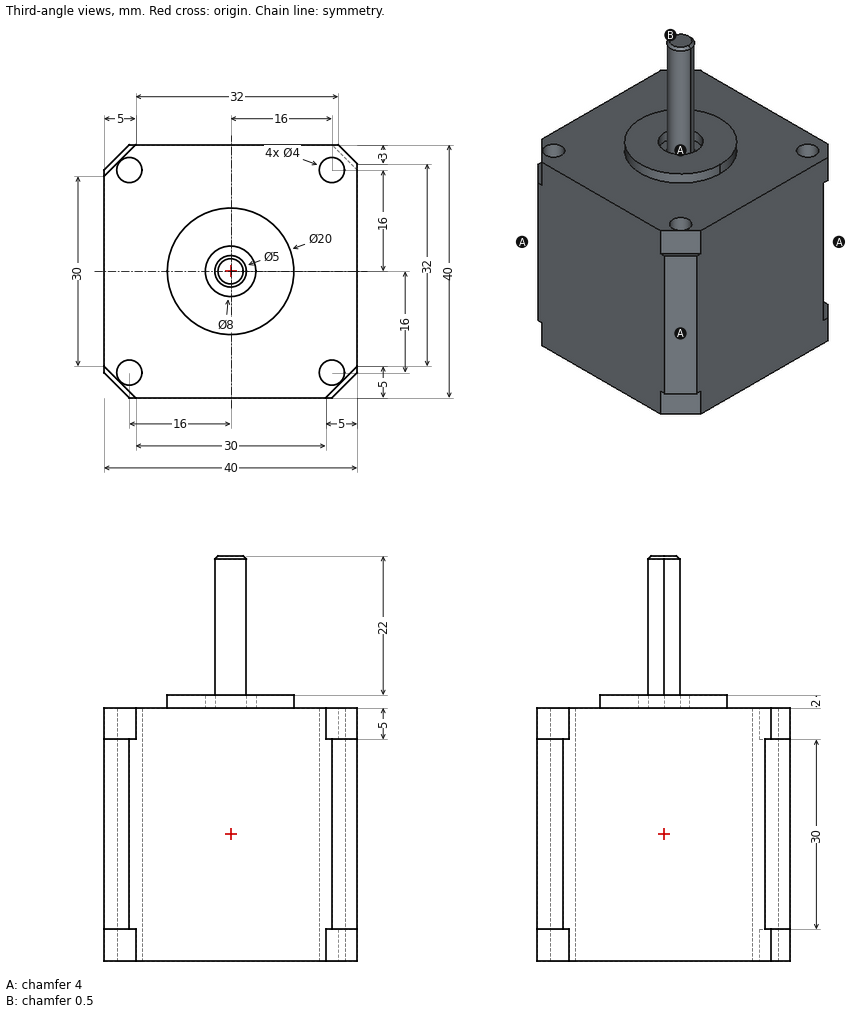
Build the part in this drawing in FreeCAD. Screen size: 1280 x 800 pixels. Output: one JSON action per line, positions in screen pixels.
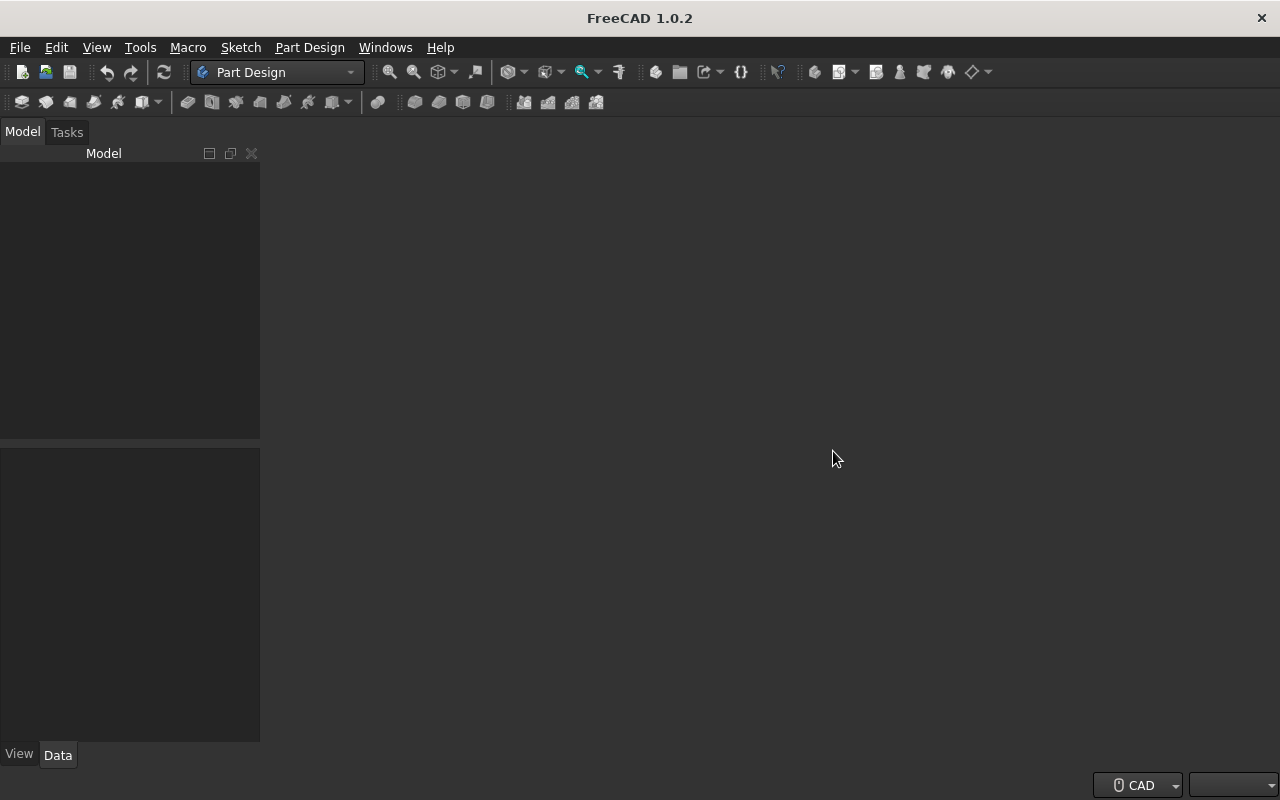
{"action": "left_click", "coordinate": [22, 72]}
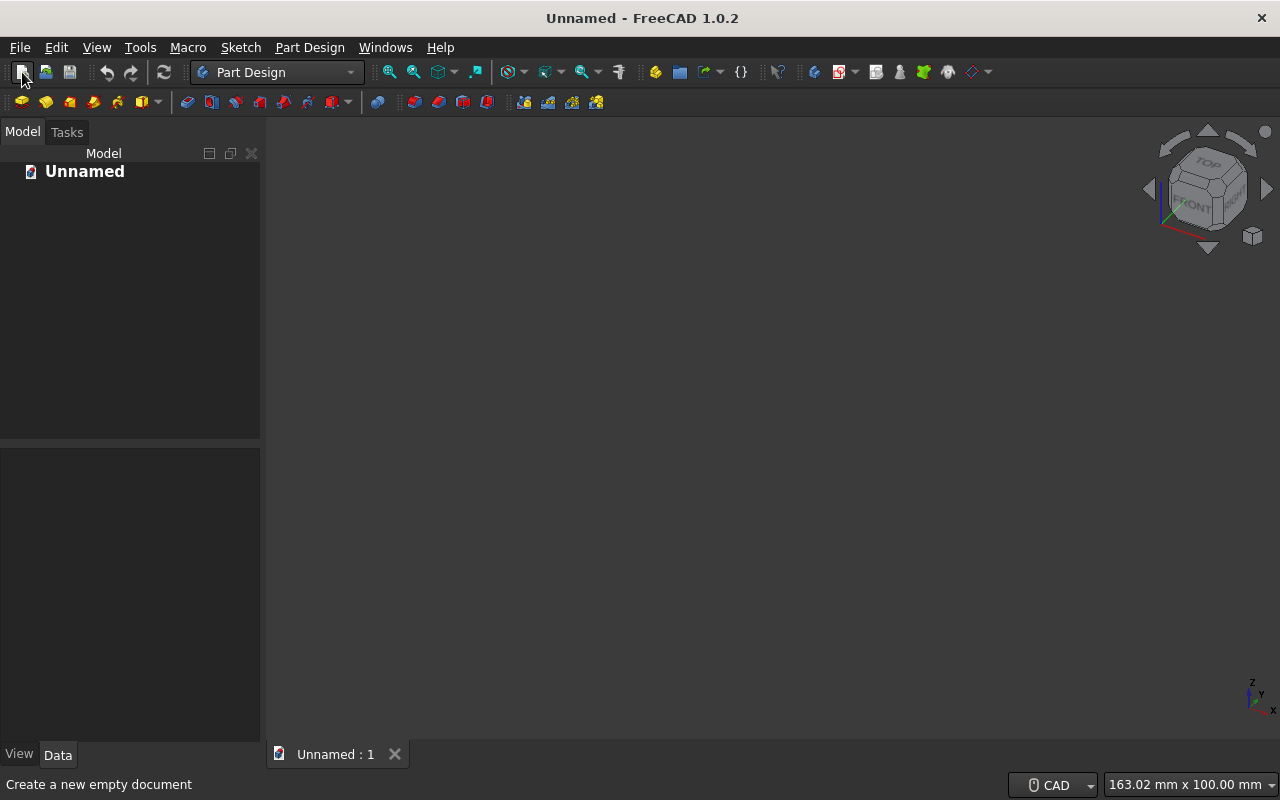
{"action": "left_click", "coordinate": [840, 72]}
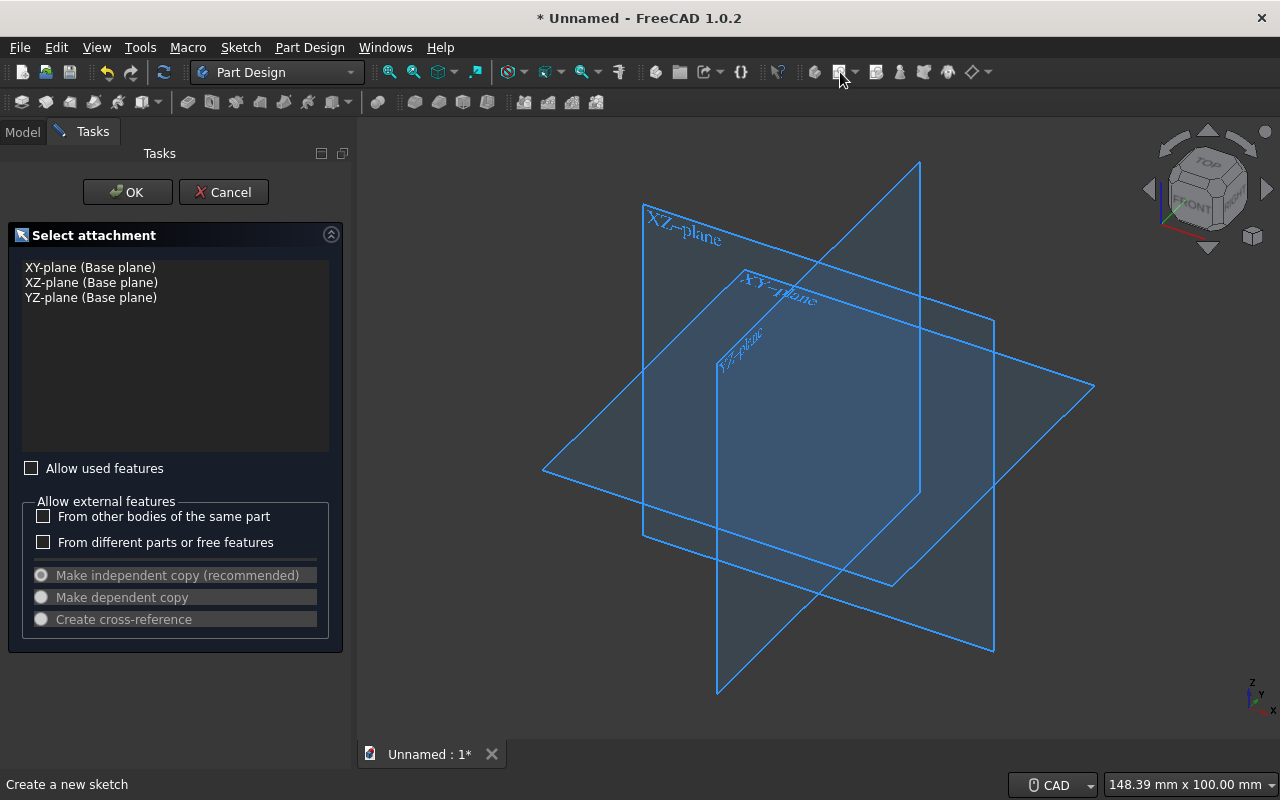
{"action": "left_click", "coordinate": [82, 268]}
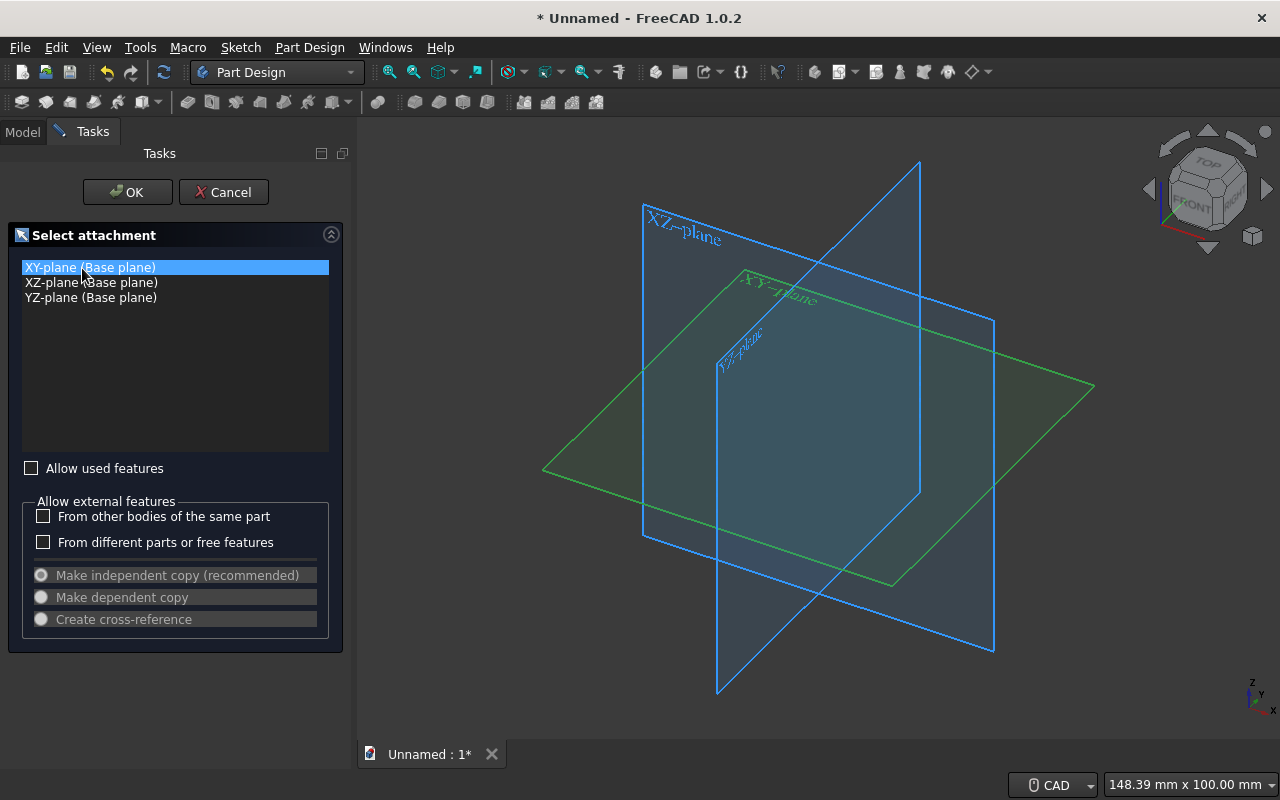
{"action": "left_click", "coordinate": [128, 192]}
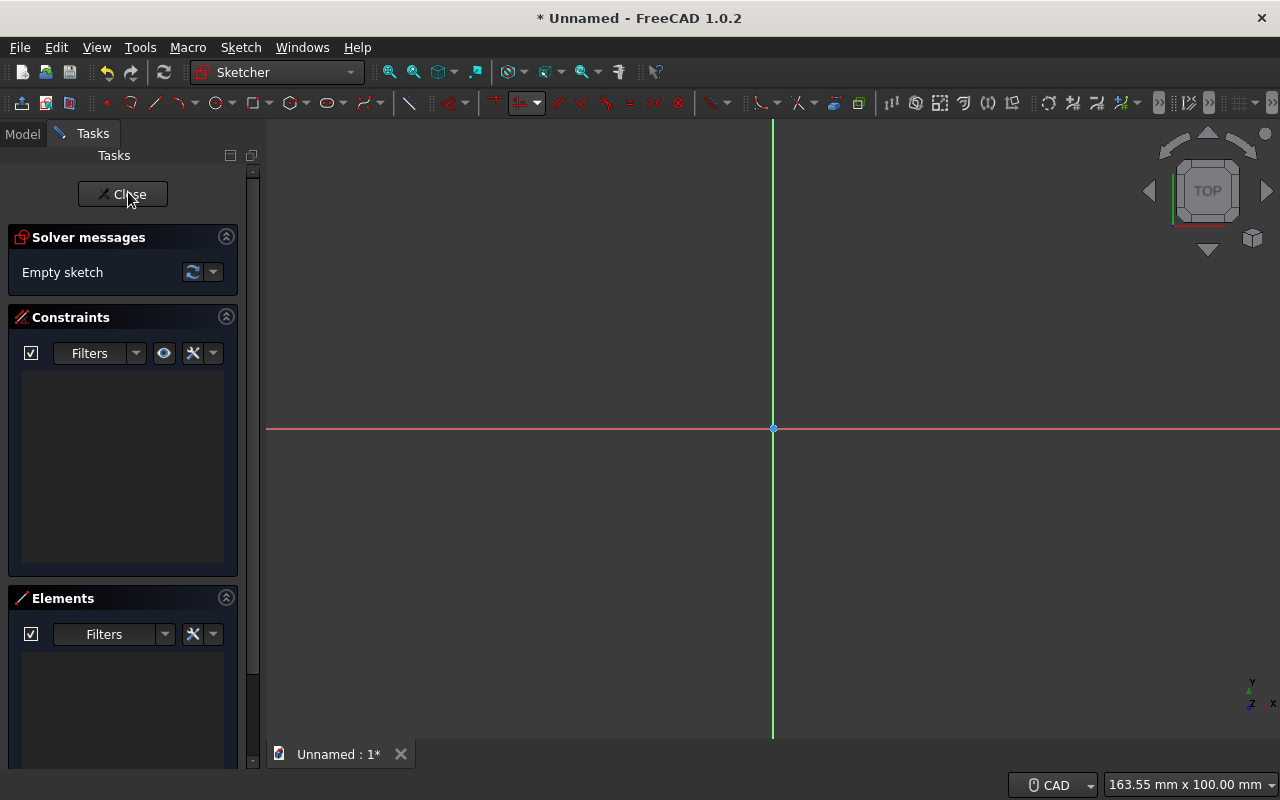
{"action": "scroll", "coordinate": [912, 429], "scroll_direction": "up", "scroll_amount": 2}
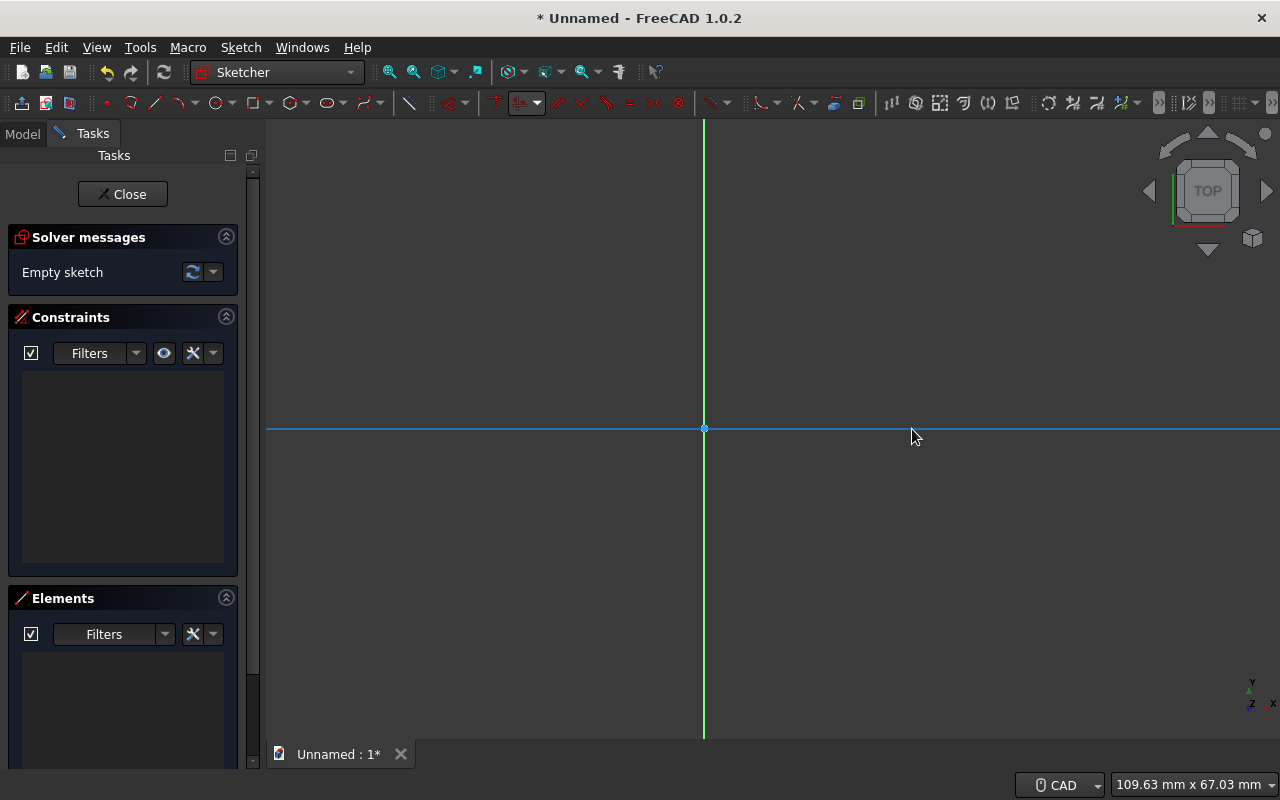
{"action": "key", "text": "g v"}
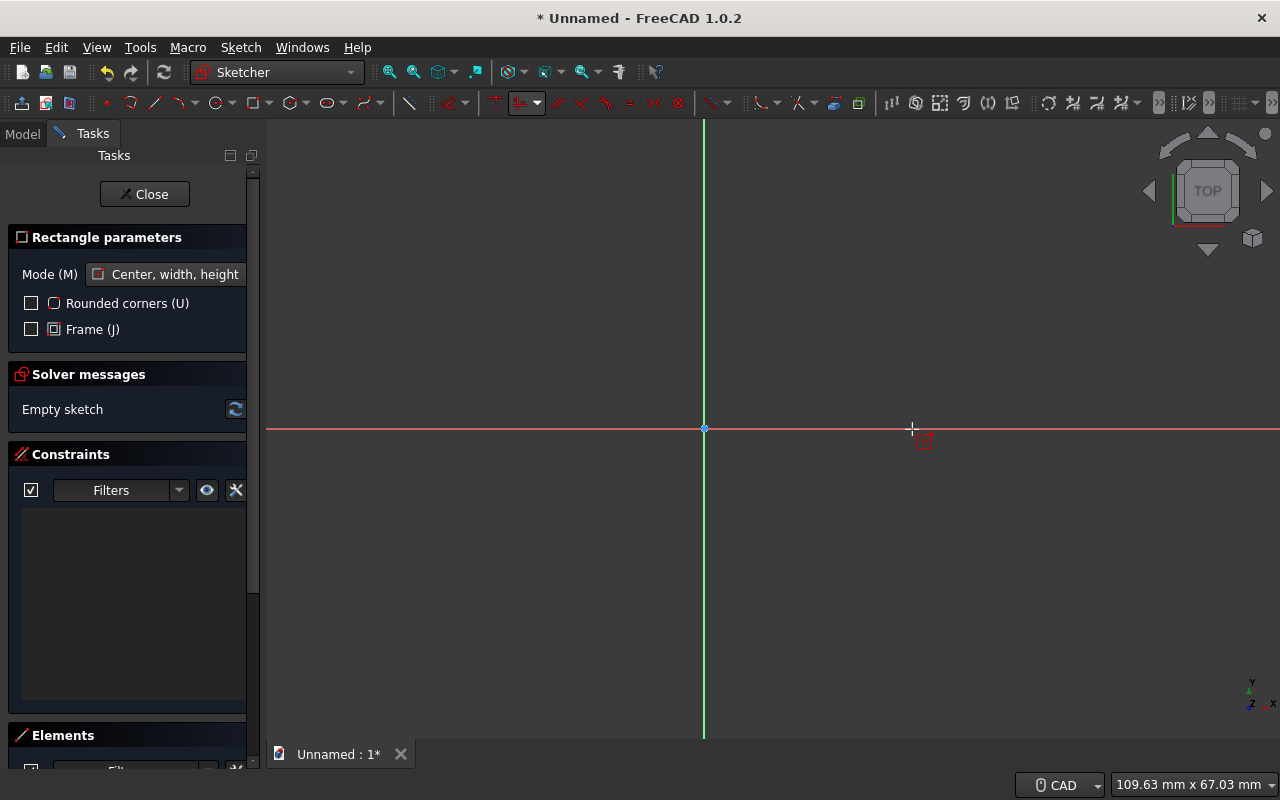
{"action": "left_click", "coordinate": [704, 429]}
{"action": "mouse_move", "coordinate": [889, 244]}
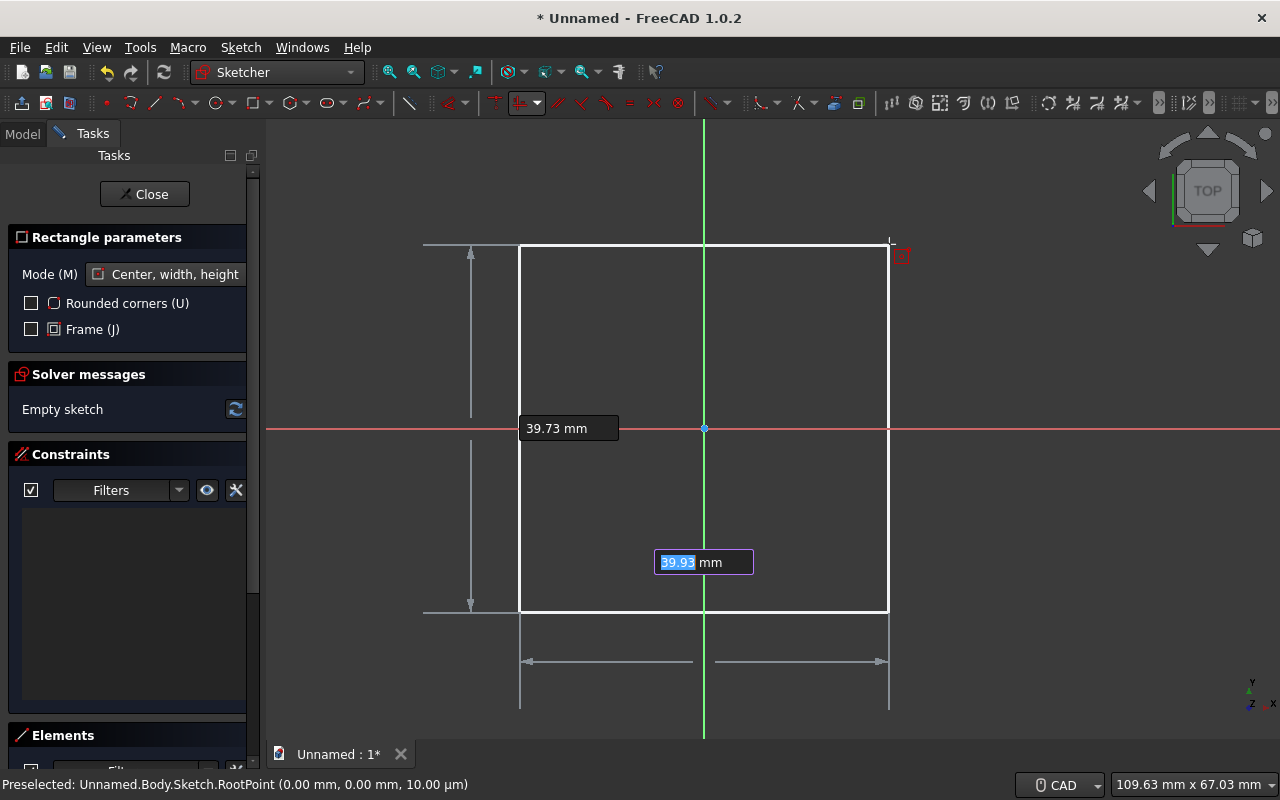
{"action": "type", "text": "40"}
{"action": "key", "text": "Tab"}
{"action": "type", "text": "40"}
{"action": "key", "text": "Return"}
{"action": "key", "text": "Escape"}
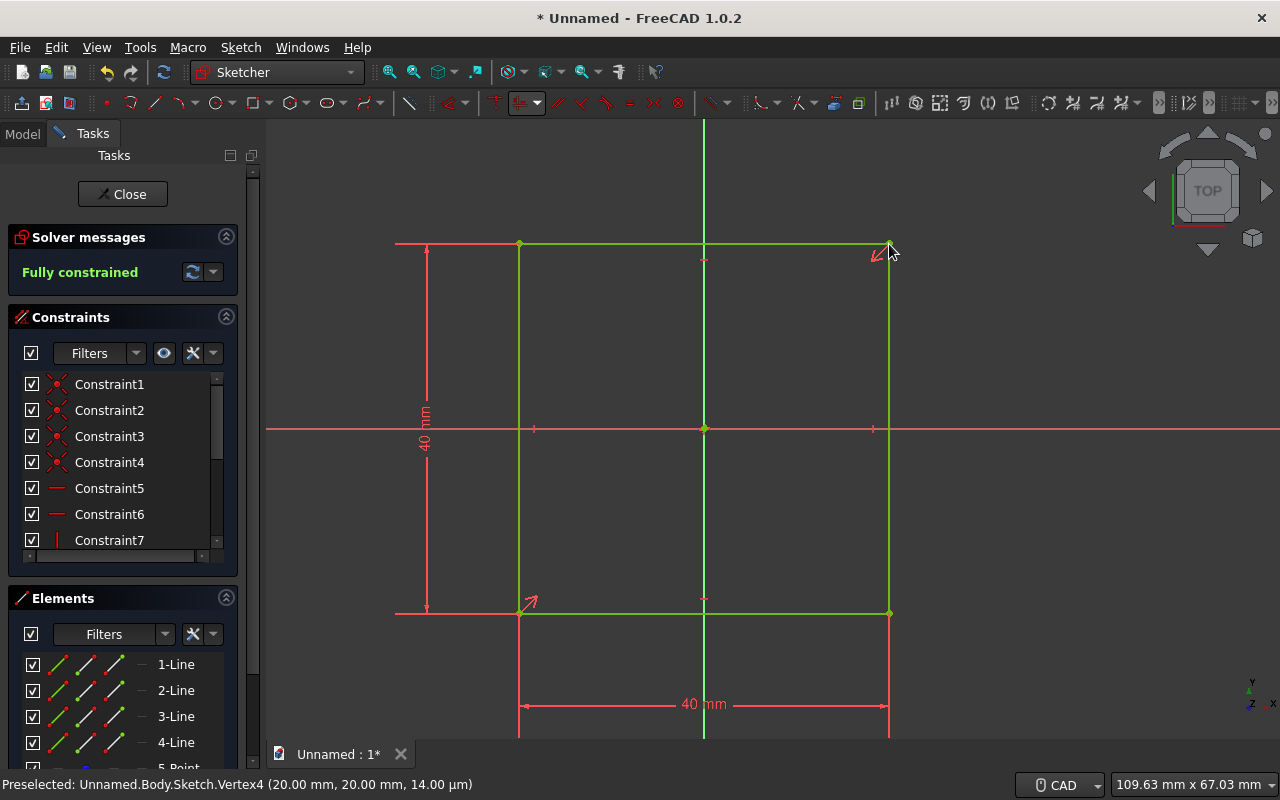
{"action": "left_click", "coordinate": [123, 194]}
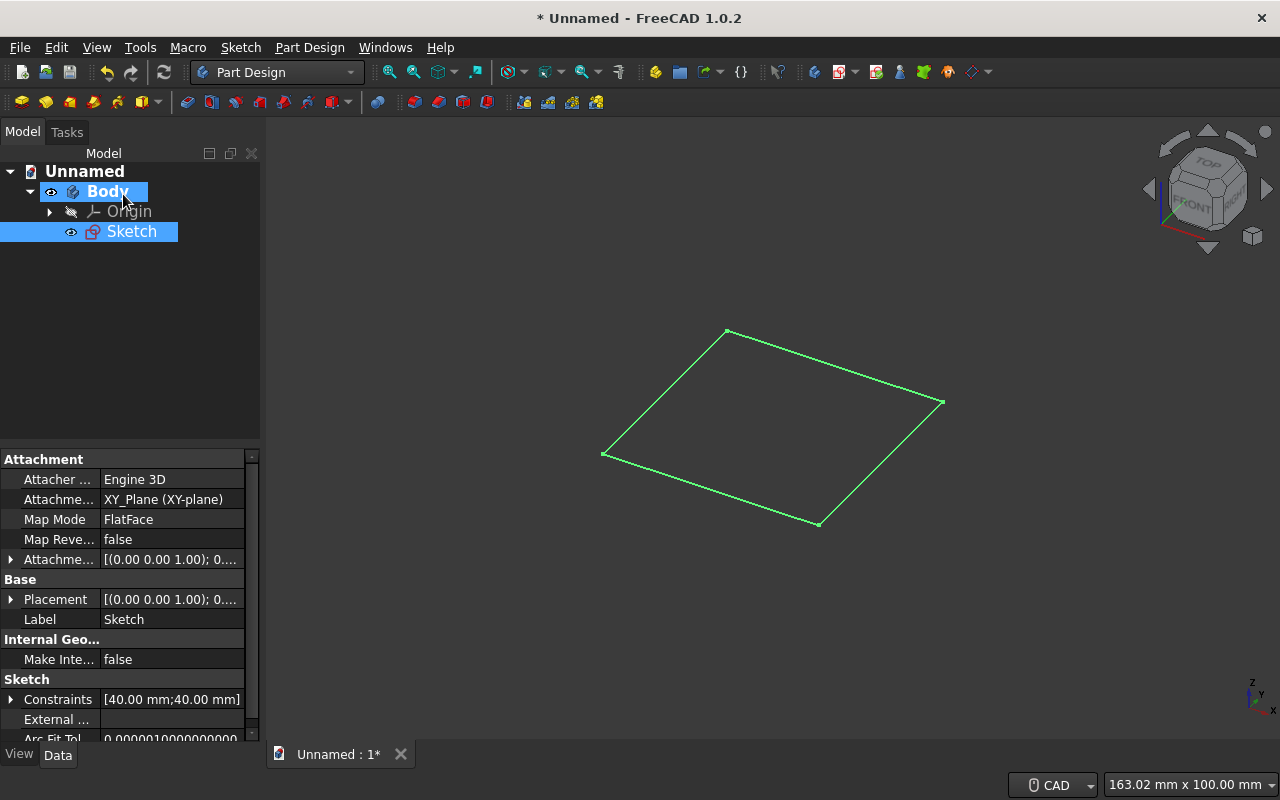
{"action": "left_click", "coordinate": [22, 102]}